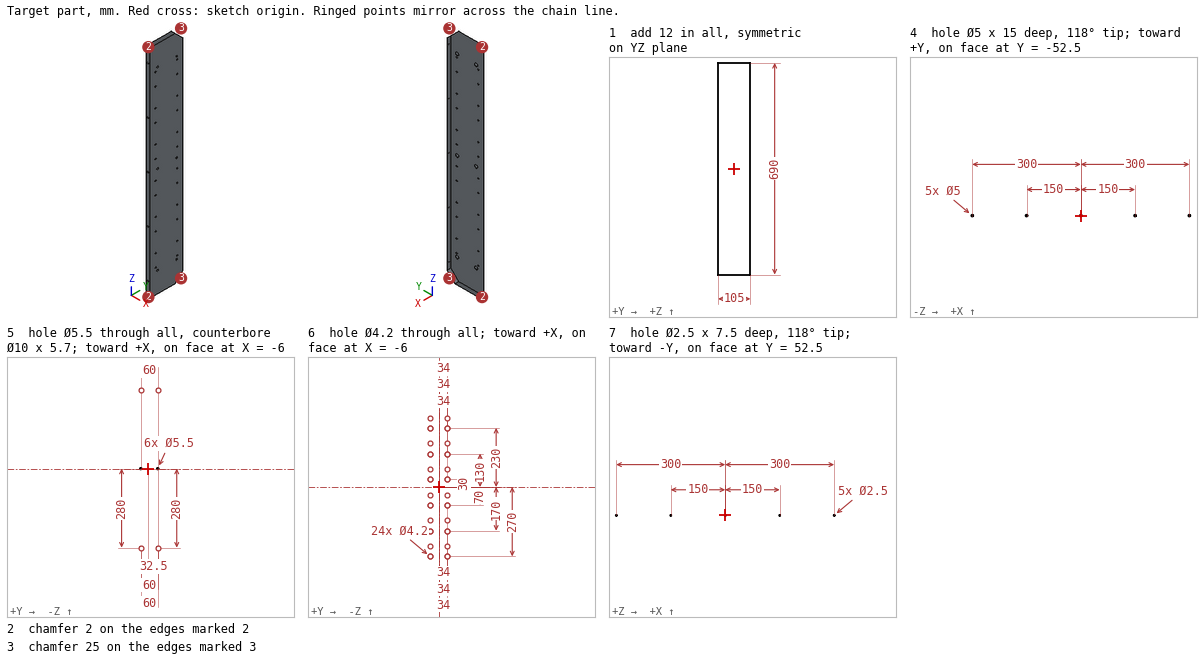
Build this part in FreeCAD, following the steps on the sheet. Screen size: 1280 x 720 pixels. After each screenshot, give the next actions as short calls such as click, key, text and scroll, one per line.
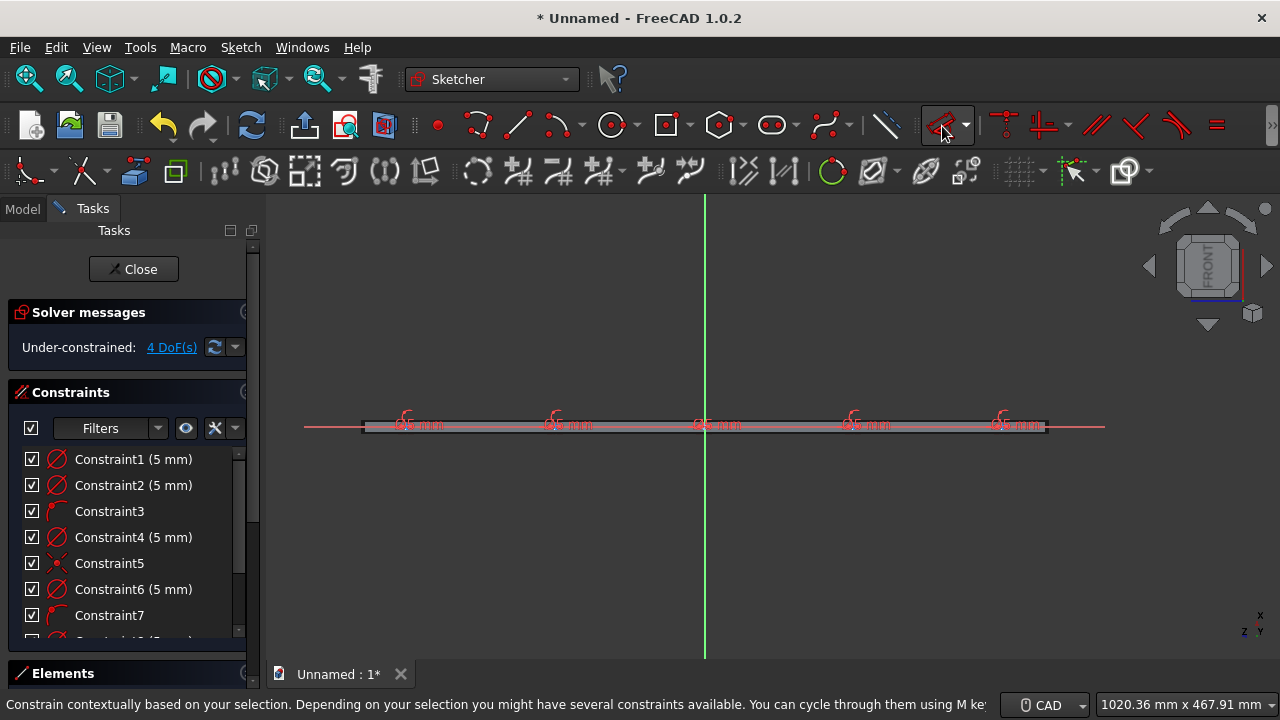
click(407, 427)
click(556, 461)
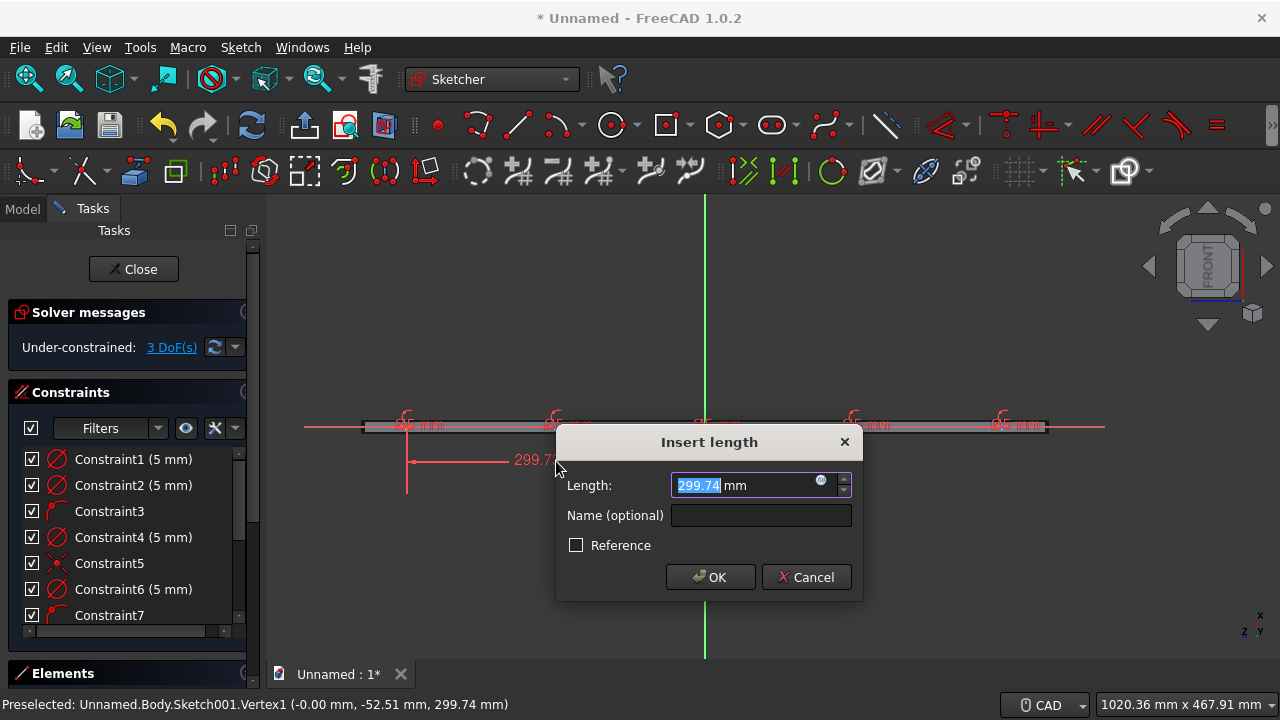
text(300)
key(Return)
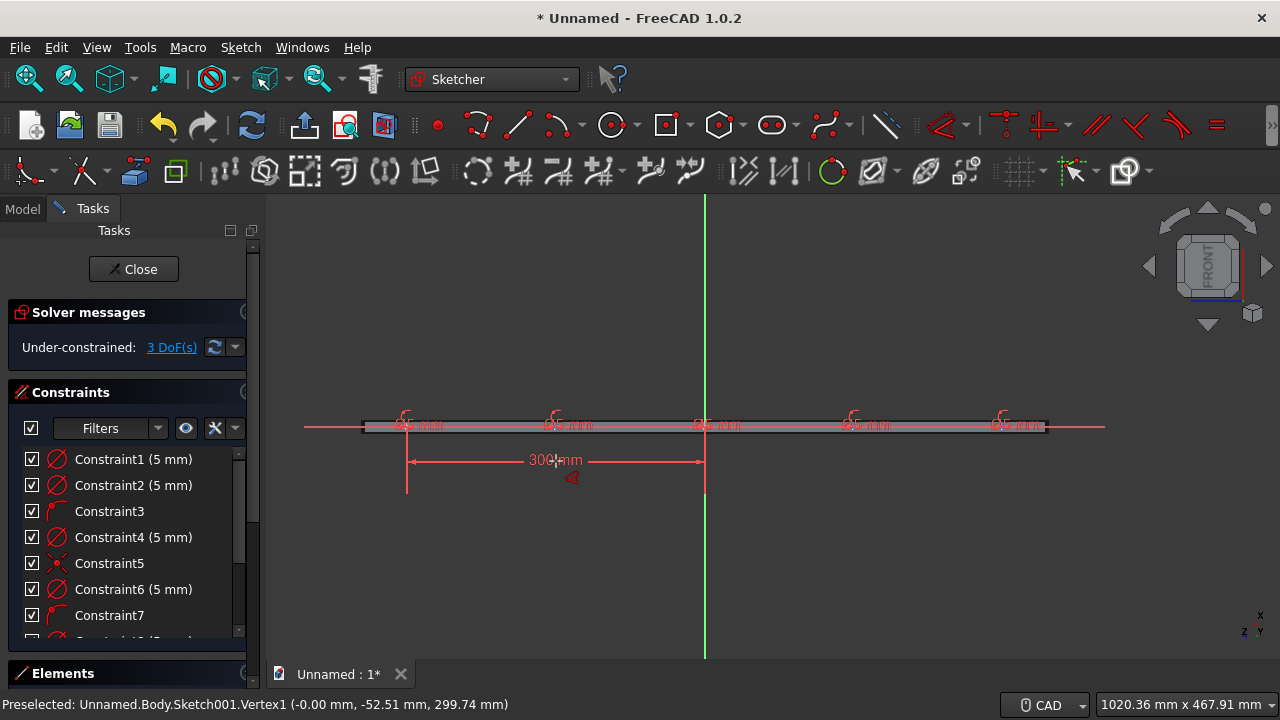
click(556, 427)
click(630, 461)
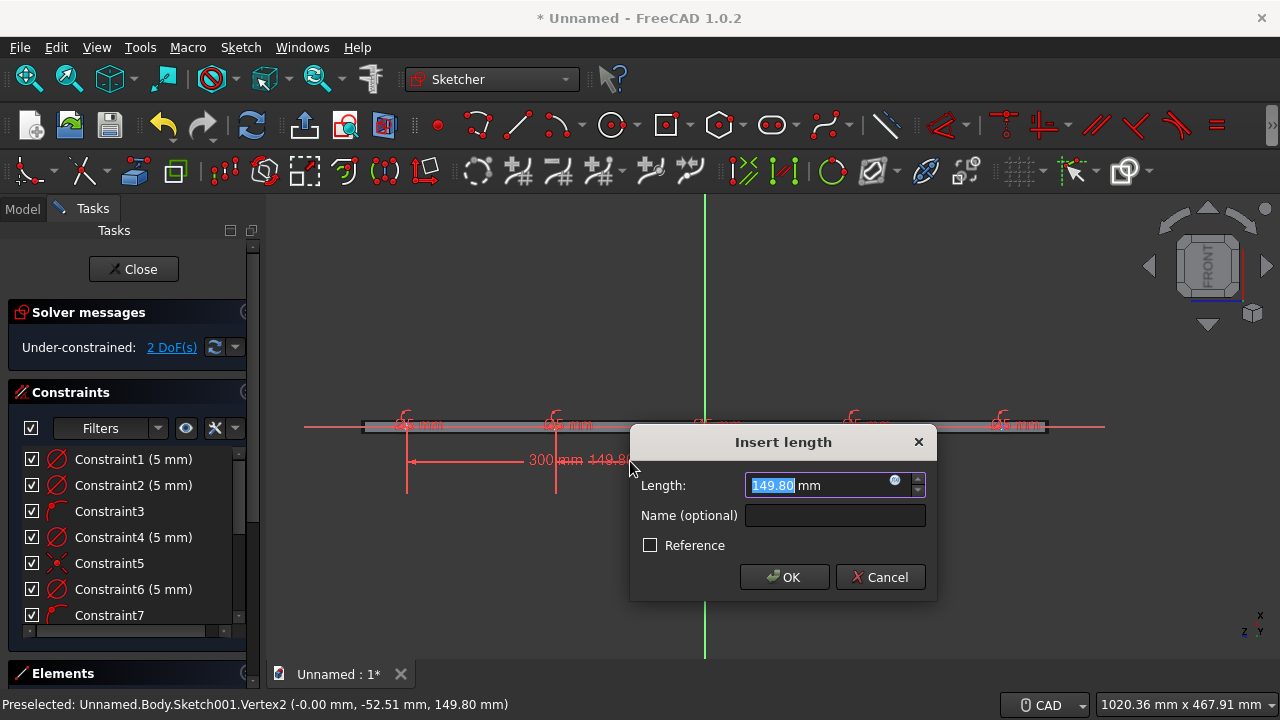
text(150)
key(Return)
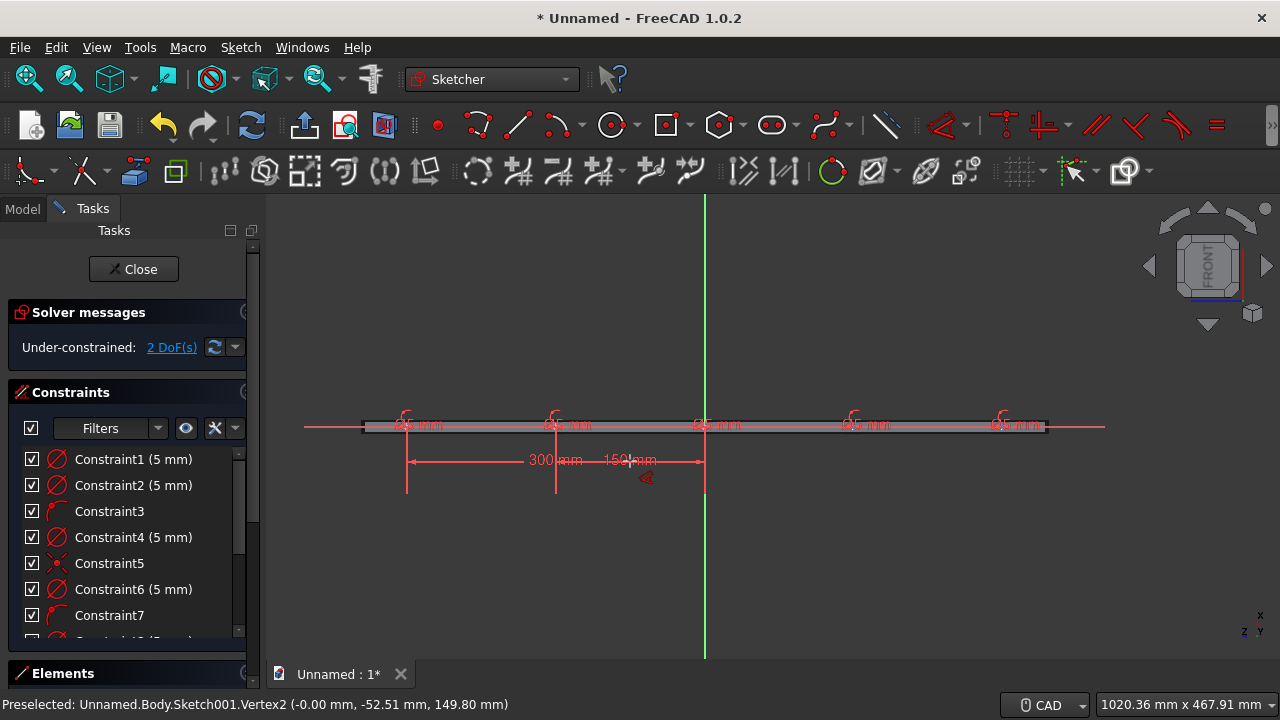
click(854, 427)
click(779, 461)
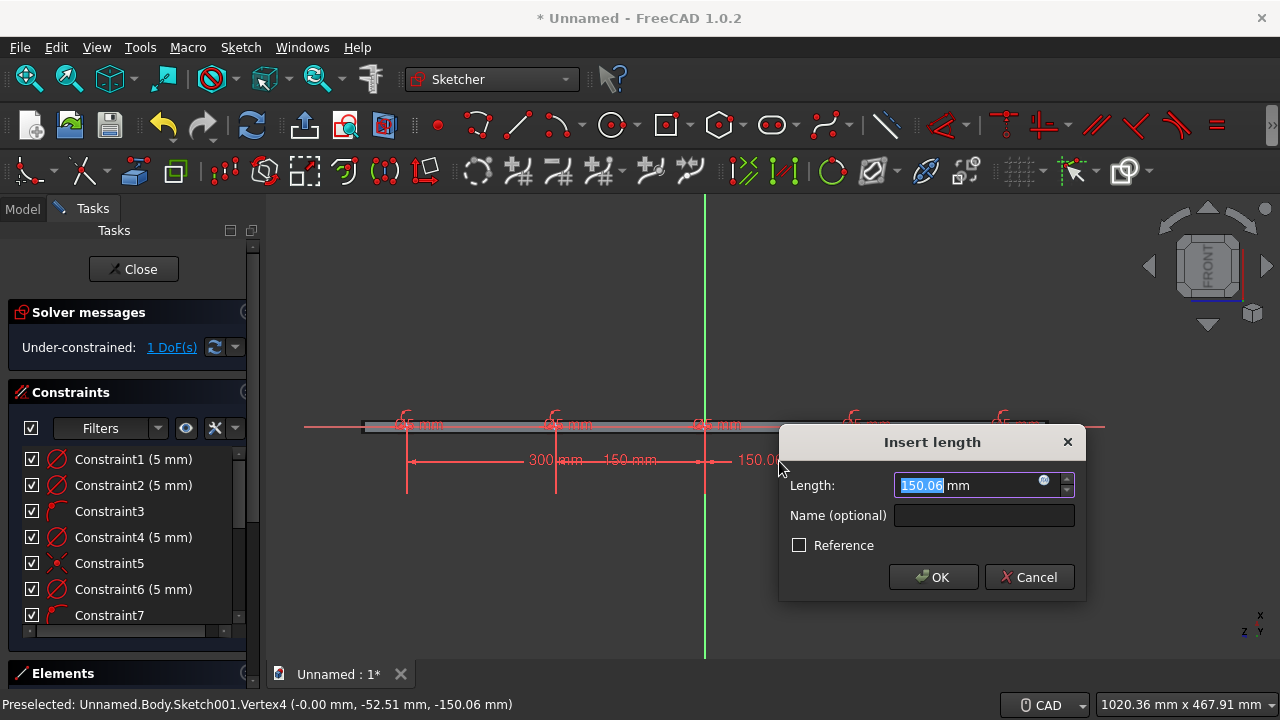
text(150)
key(Return)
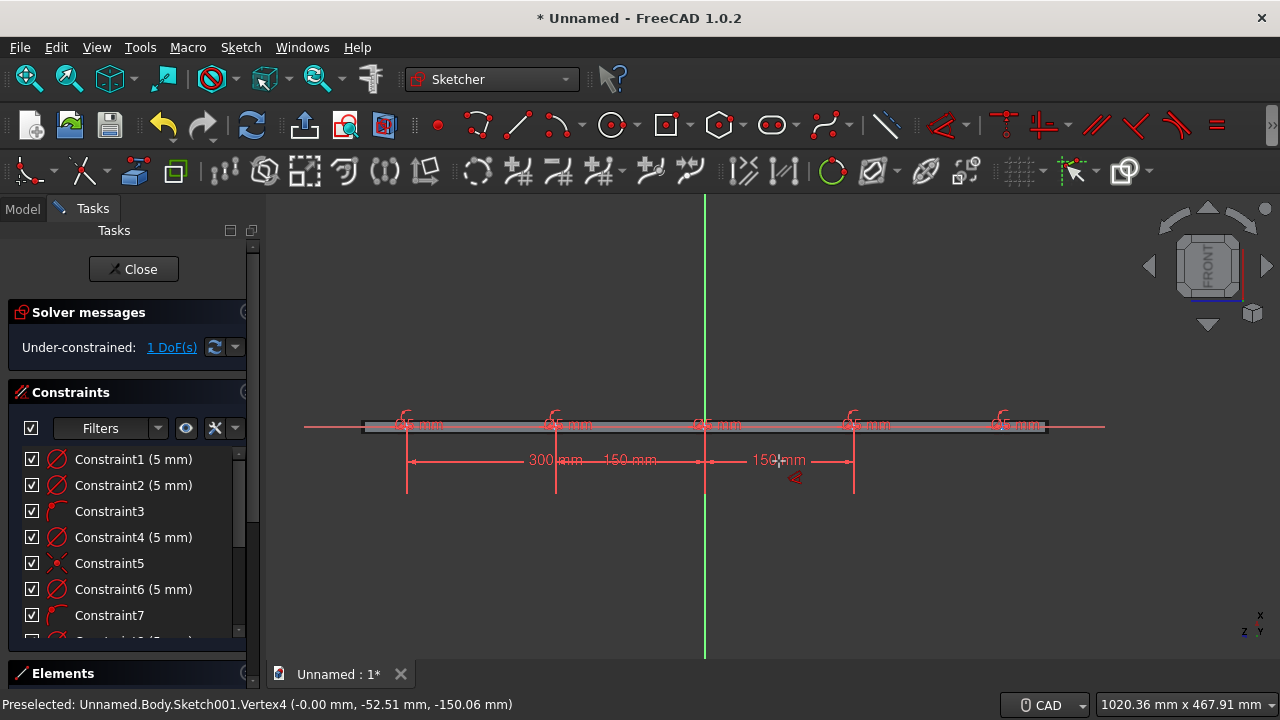
click(1003, 427)
click(854, 461)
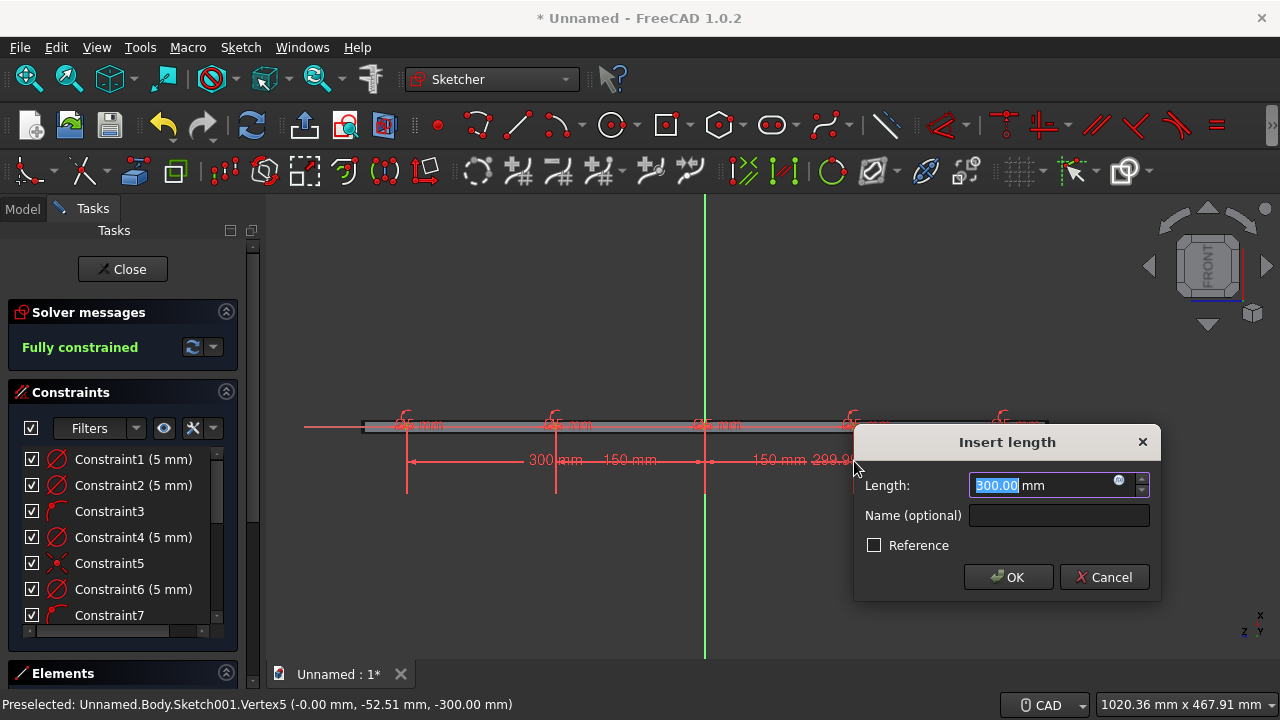
text(300)
key(Return)
key(Escape)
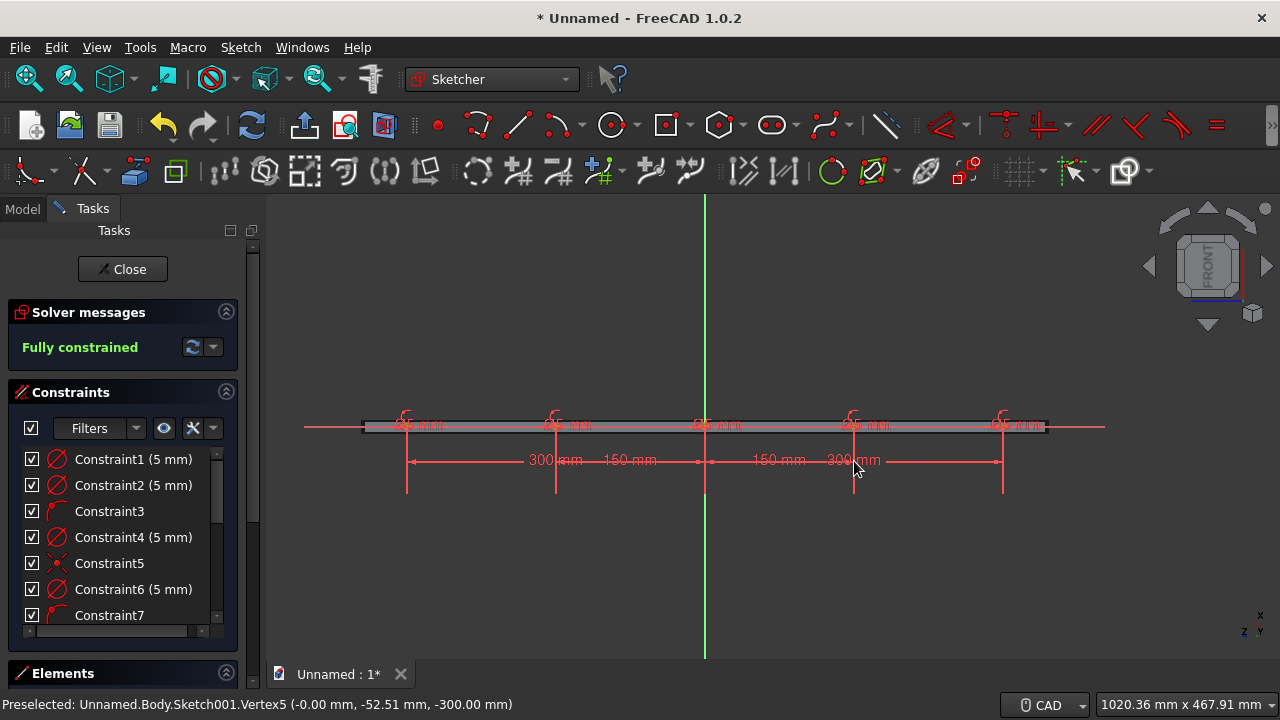
click(123, 269)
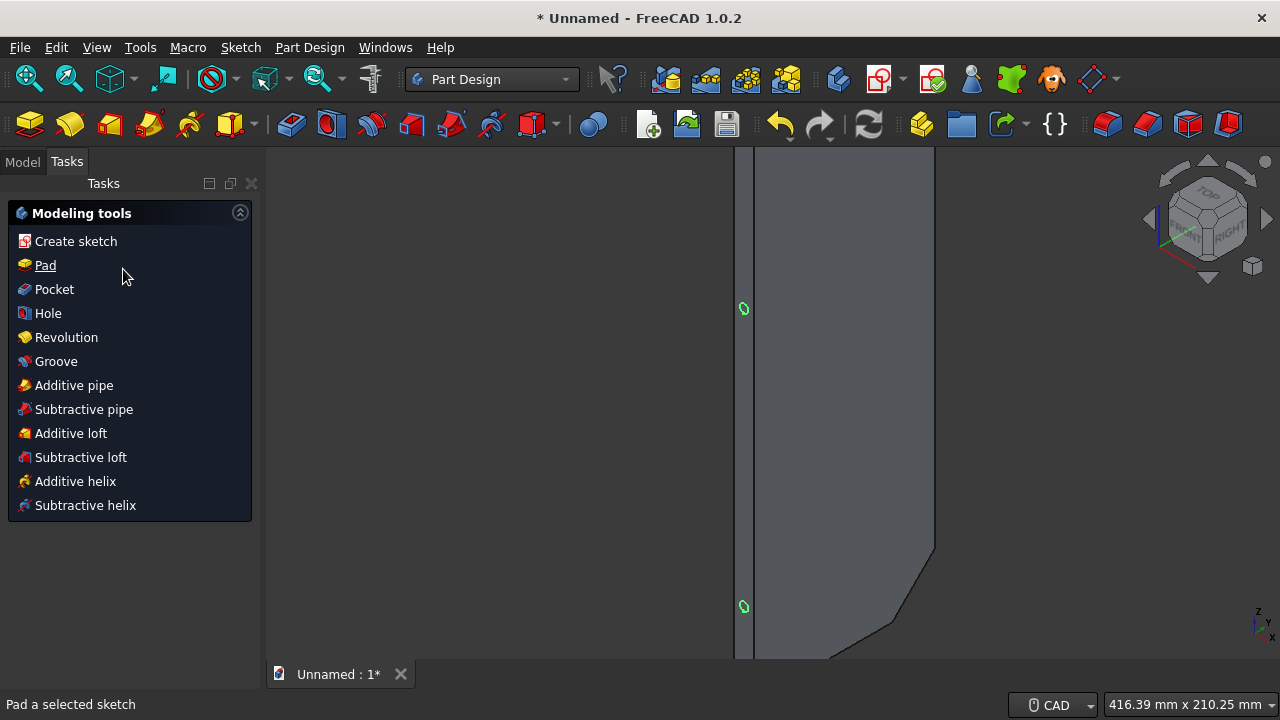
click(332, 124)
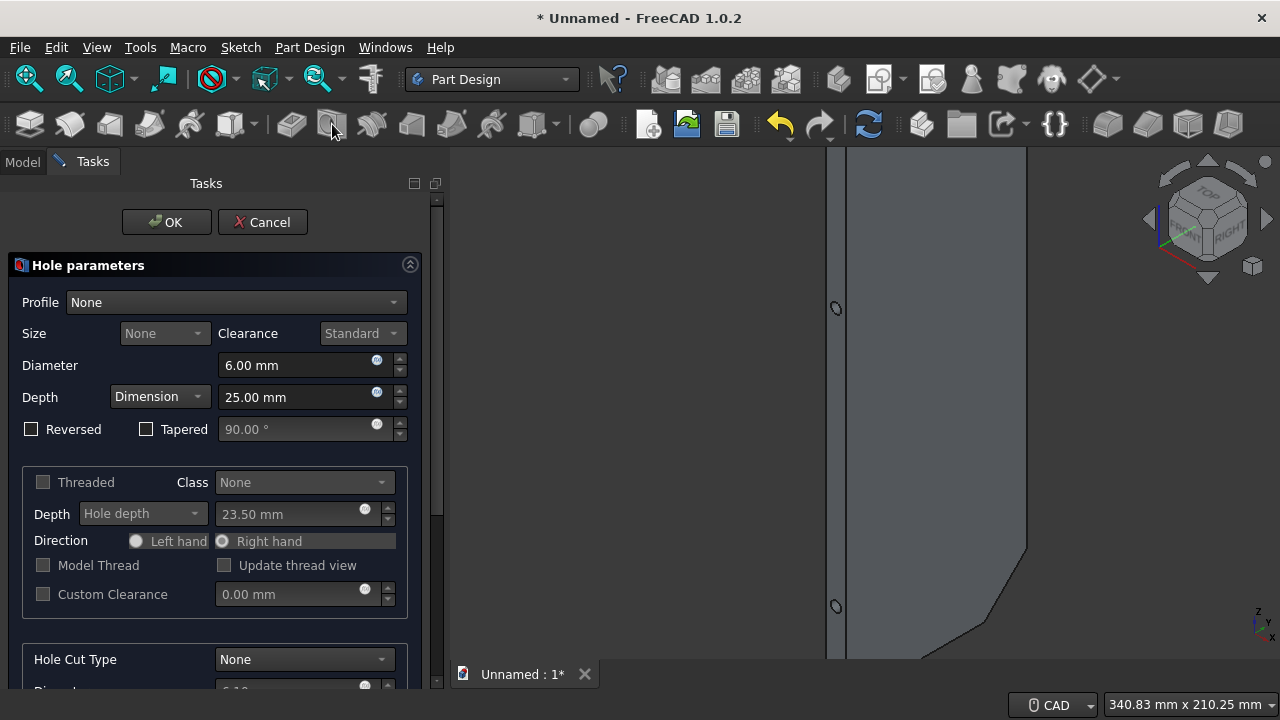
triple_click(305, 365)